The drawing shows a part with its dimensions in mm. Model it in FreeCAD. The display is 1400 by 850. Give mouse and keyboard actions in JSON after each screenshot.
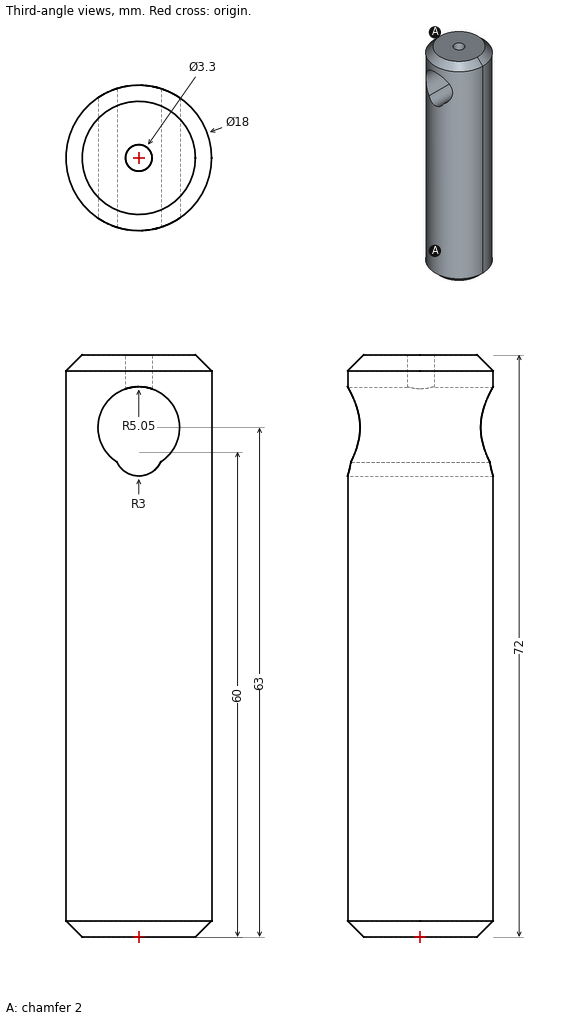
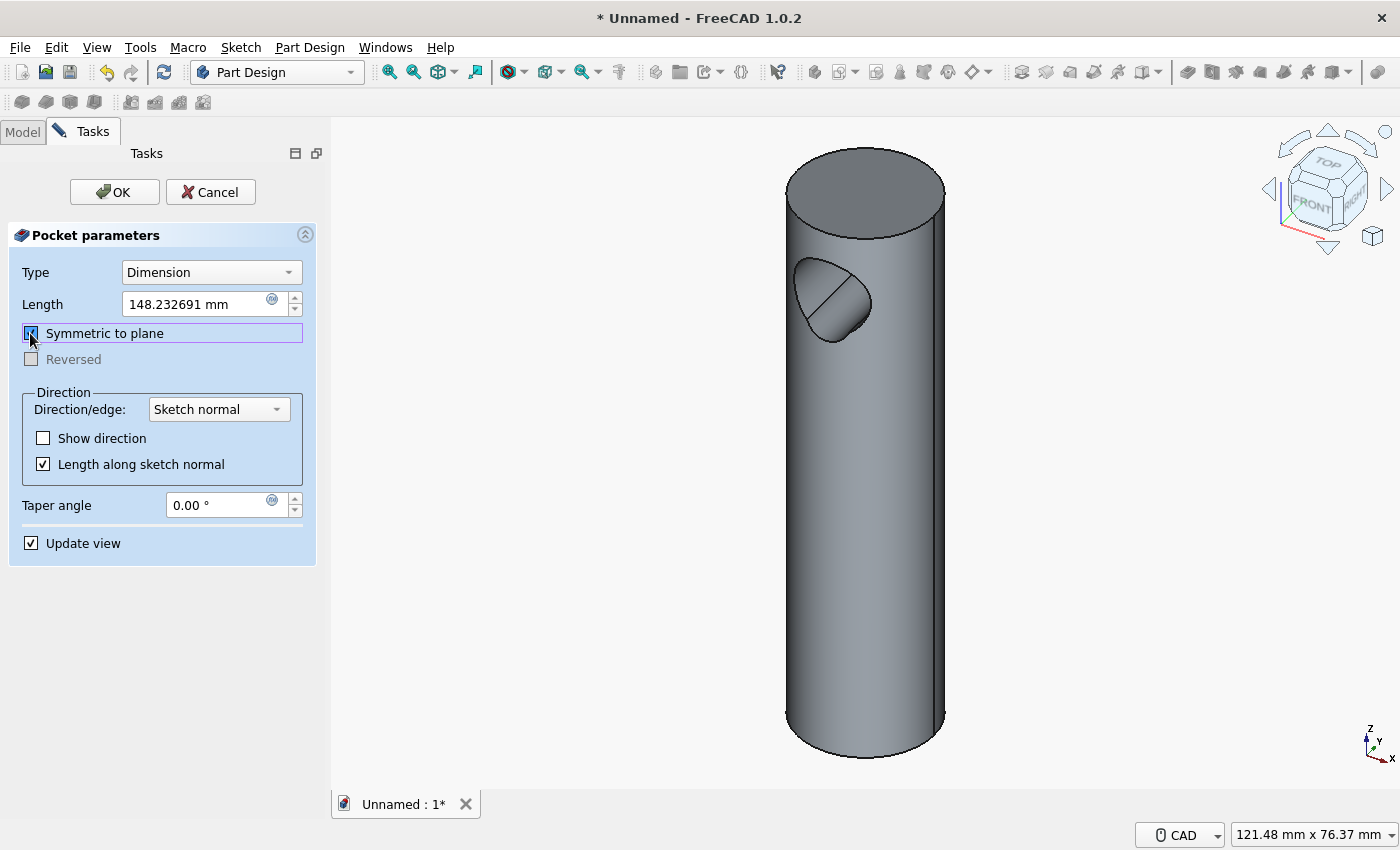
{"action": "left_click", "coordinate": [115, 192]}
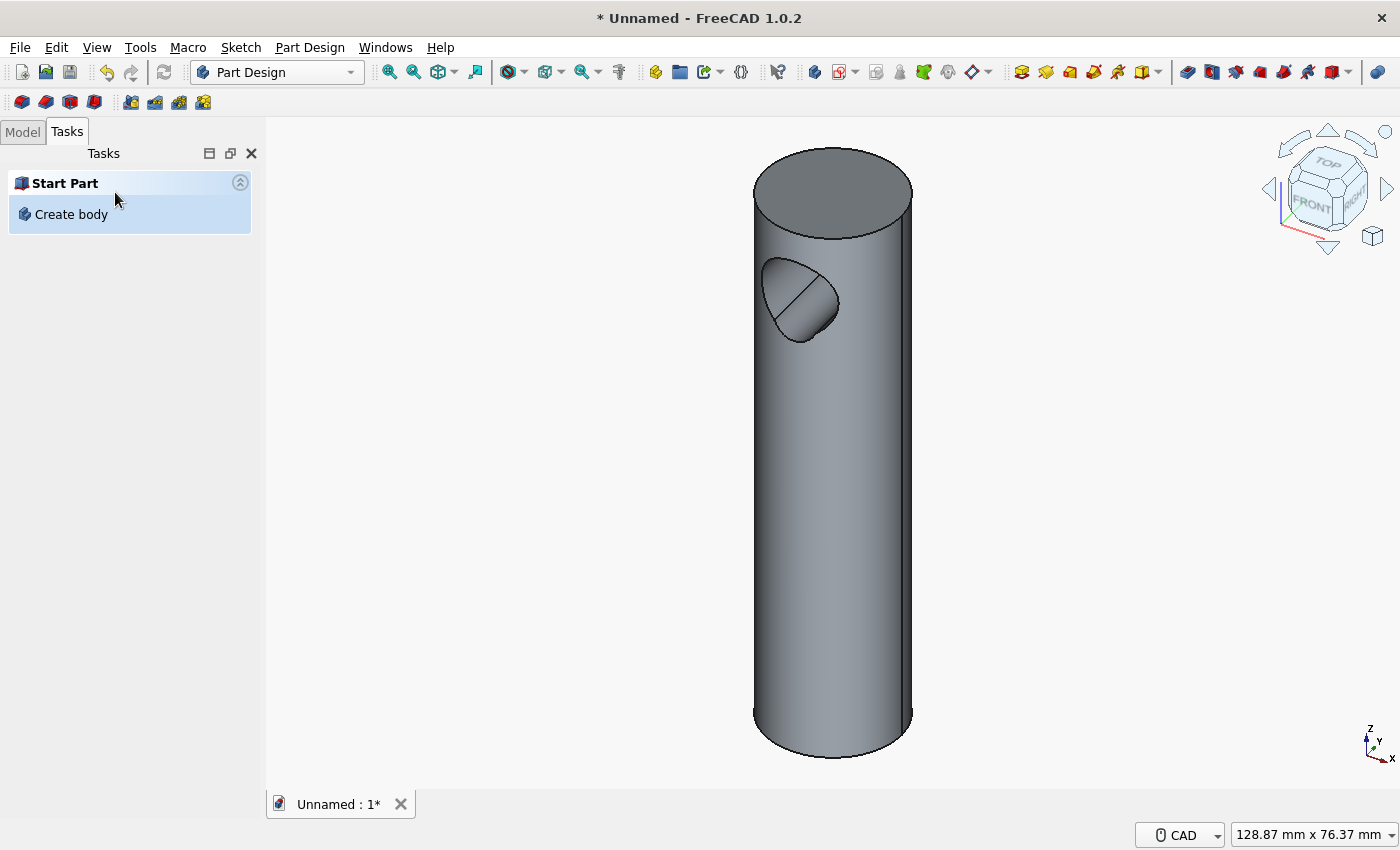
{"action": "left_click", "coordinate": [833, 193]}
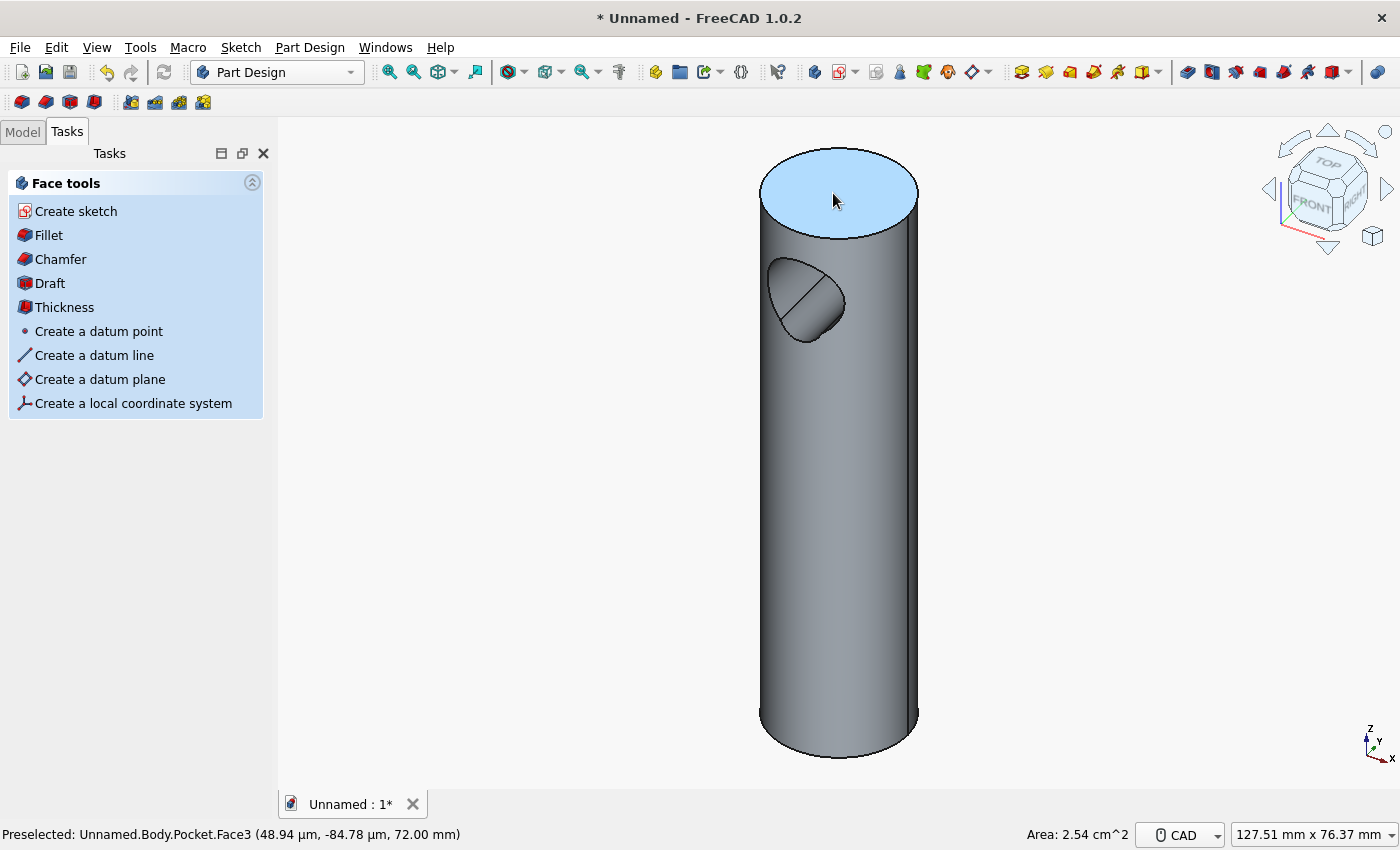
{"action": "left_click", "coordinate": [840, 72]}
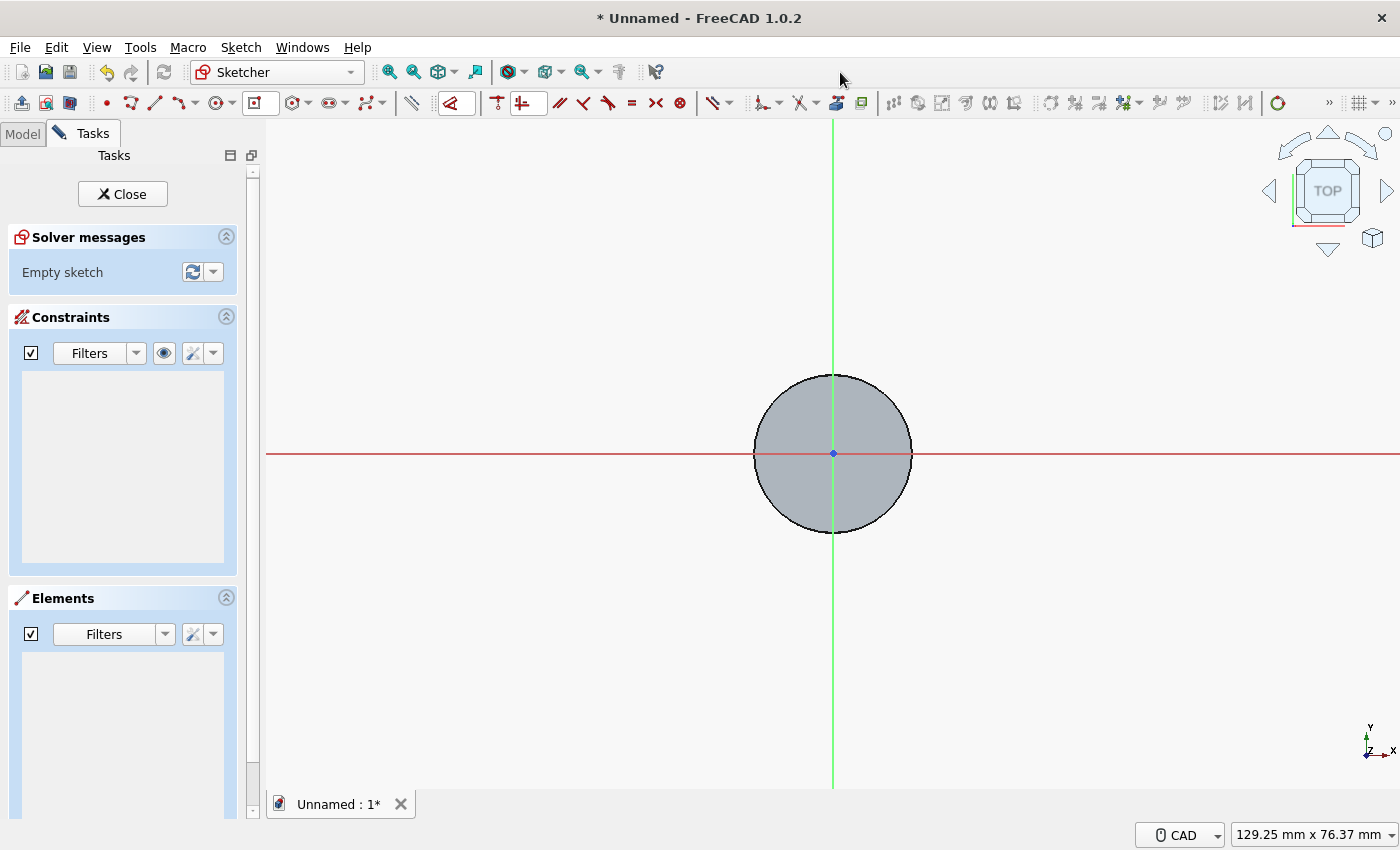
{"action": "scroll", "coordinate": [837, 454], "scroll_direction": "up", "scroll_amount": 14}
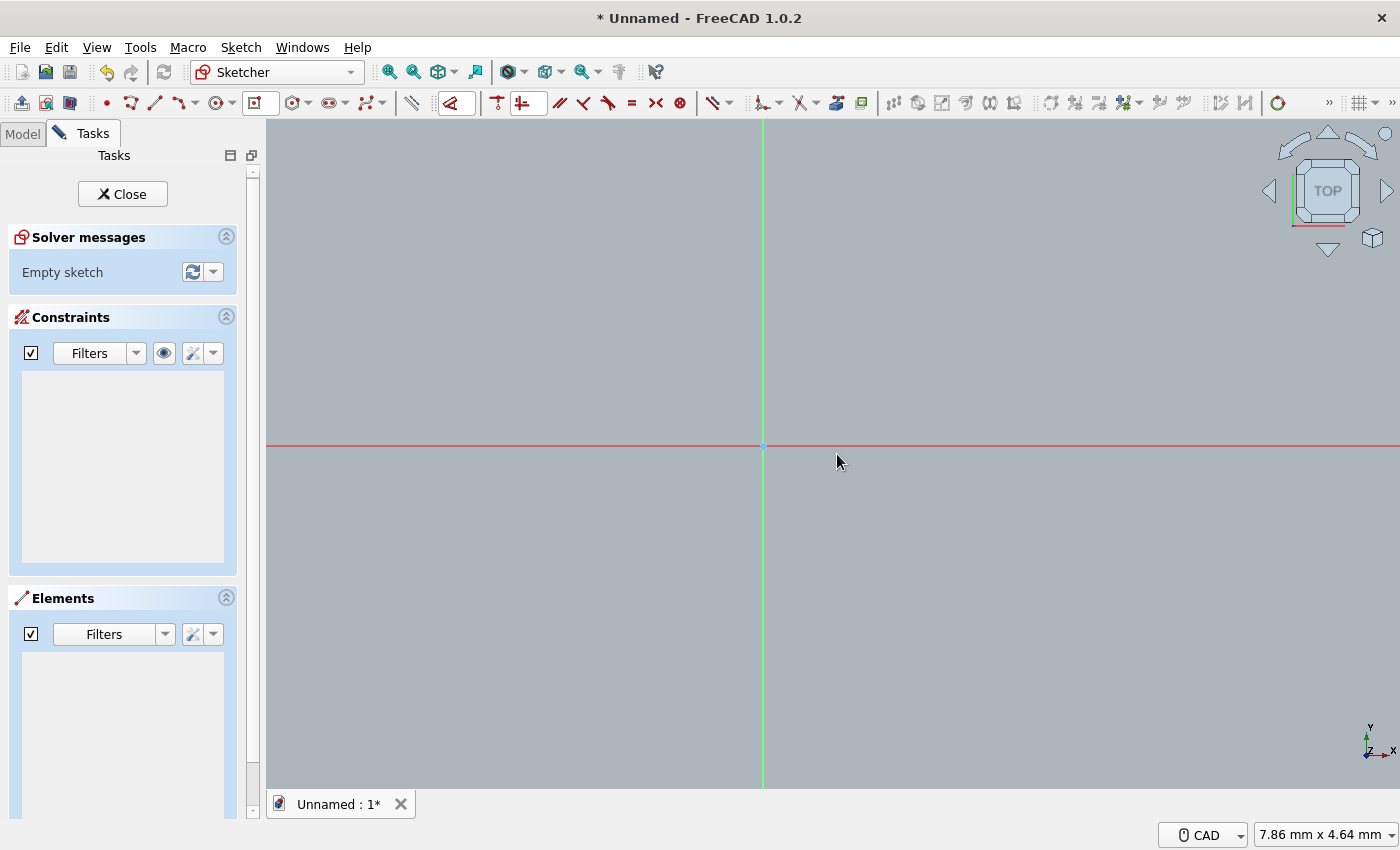
{"action": "left_click", "coordinate": [216, 104]}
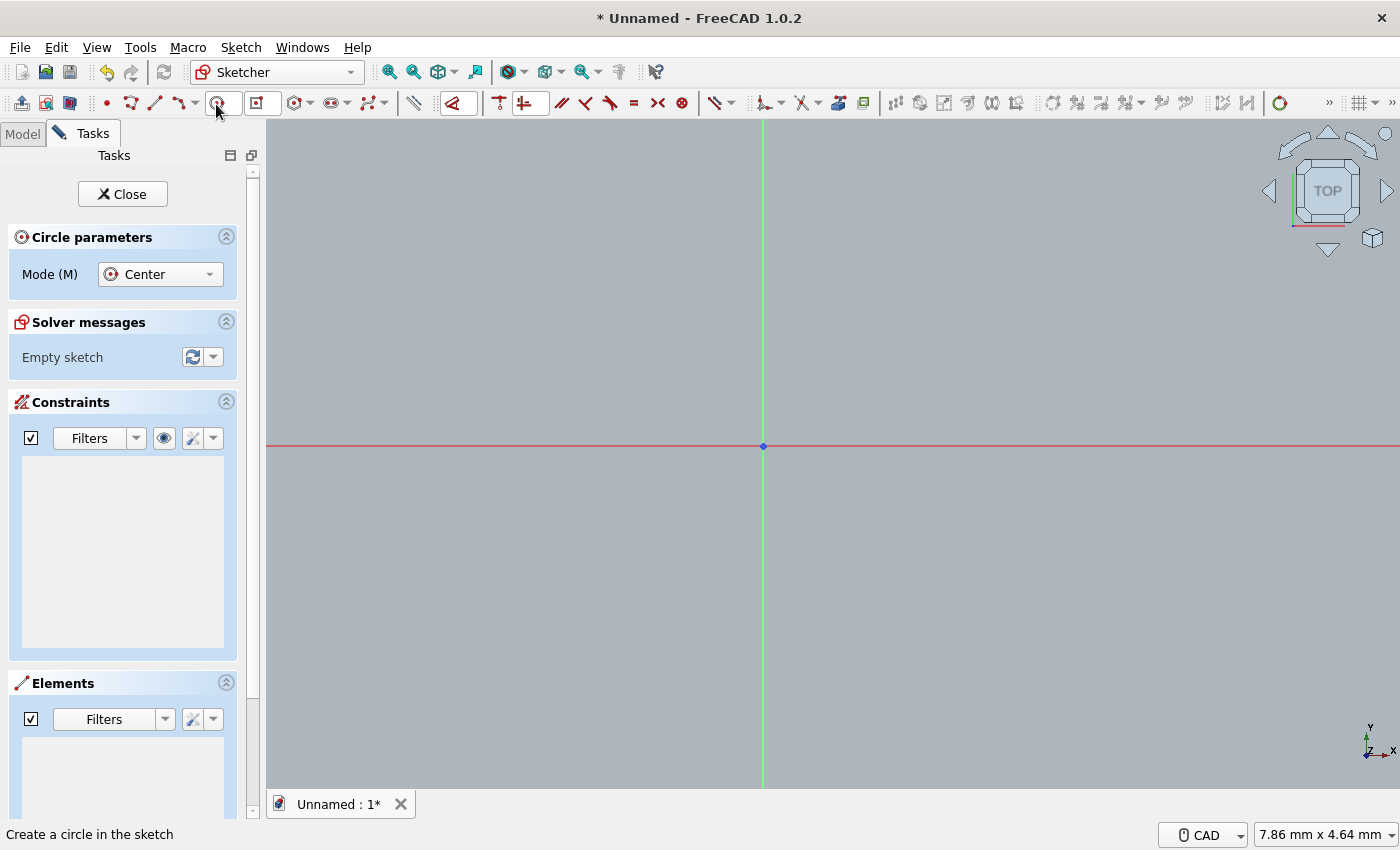
{"action": "left_click", "coordinate": [763, 446]}
{"action": "mouse_move", "coordinate": [932, 278]}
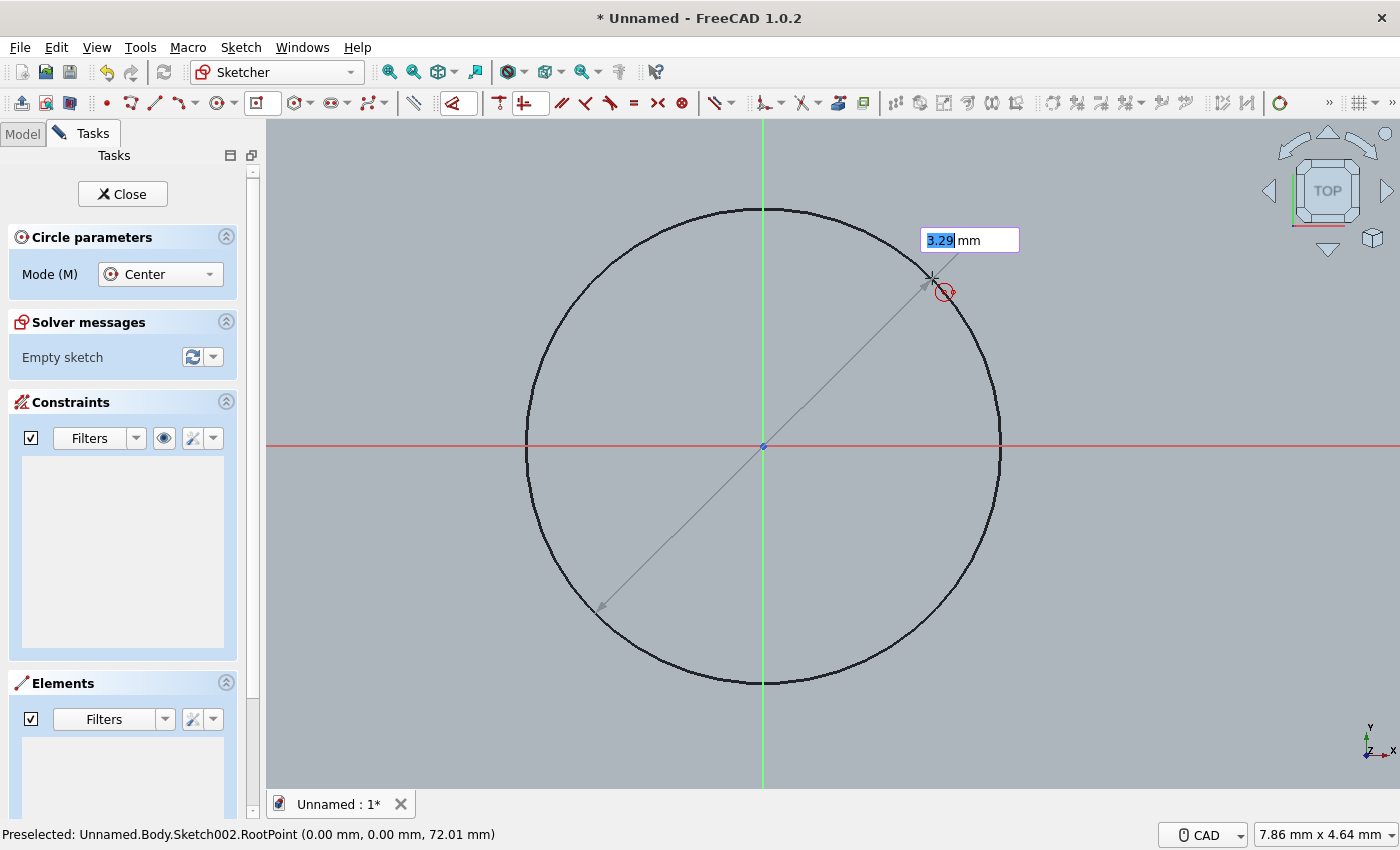
{"action": "type", "text": "3.3"}
{"action": "key", "text": "Return"}
{"action": "key", "text": "Escape"}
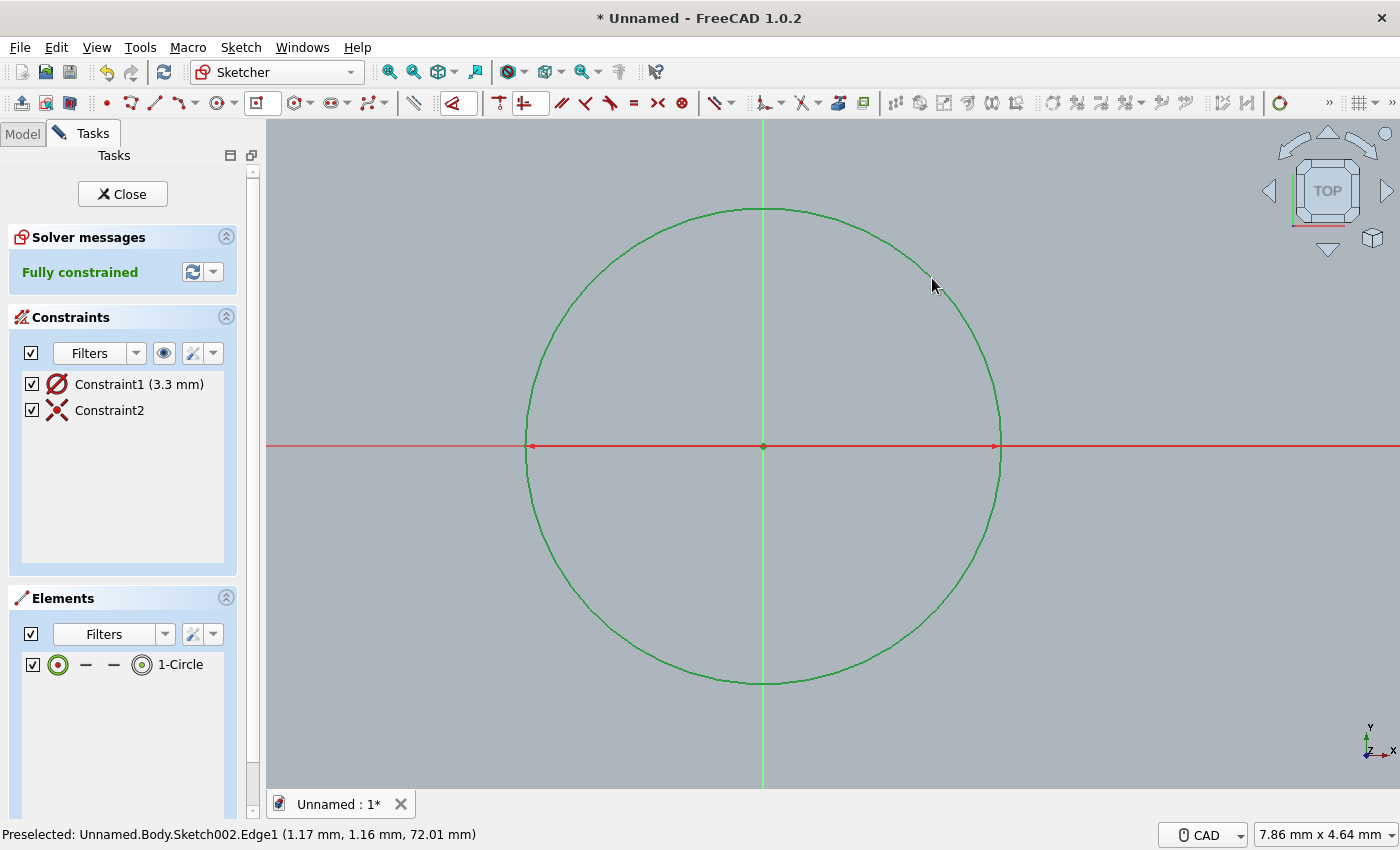
{"action": "left_click", "coordinate": [123, 194]}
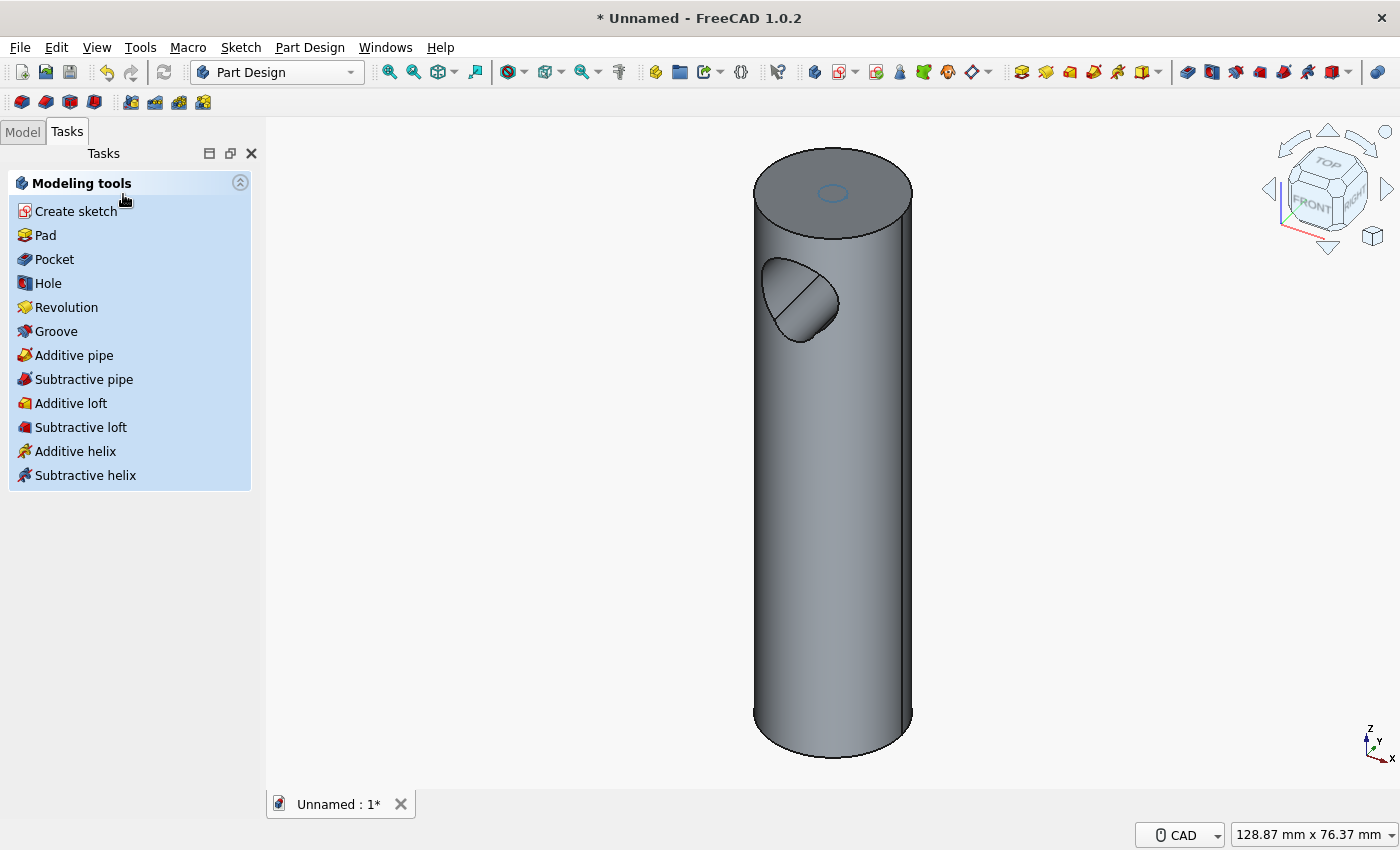
{"action": "left_click", "coordinate": [1188, 72]}